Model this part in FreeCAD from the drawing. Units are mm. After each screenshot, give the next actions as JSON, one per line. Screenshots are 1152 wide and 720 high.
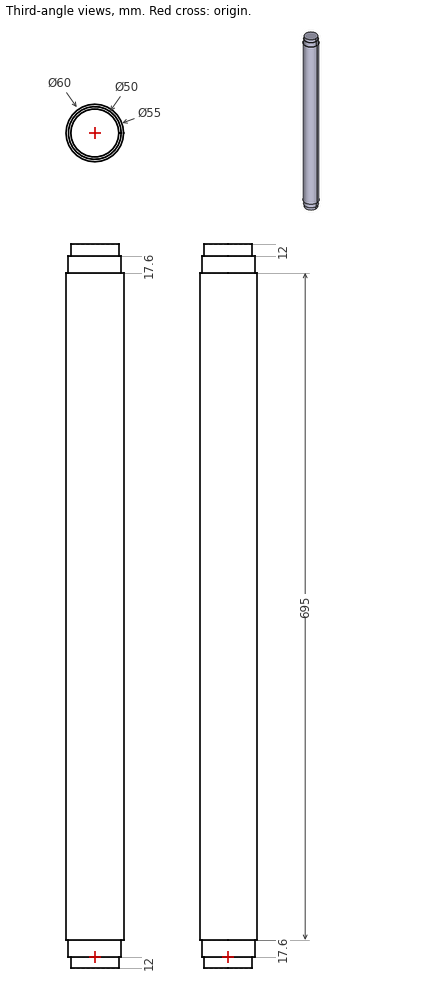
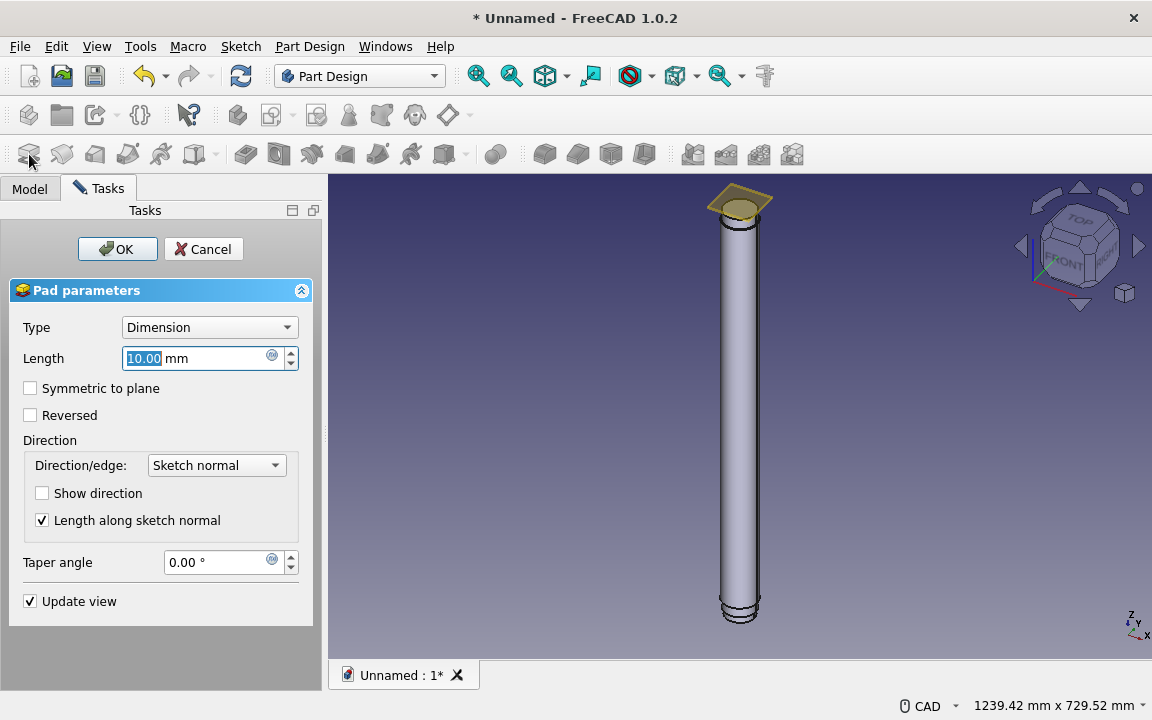
{"action": "type", "text": "12"}
{"action": "key", "text": "Tab"}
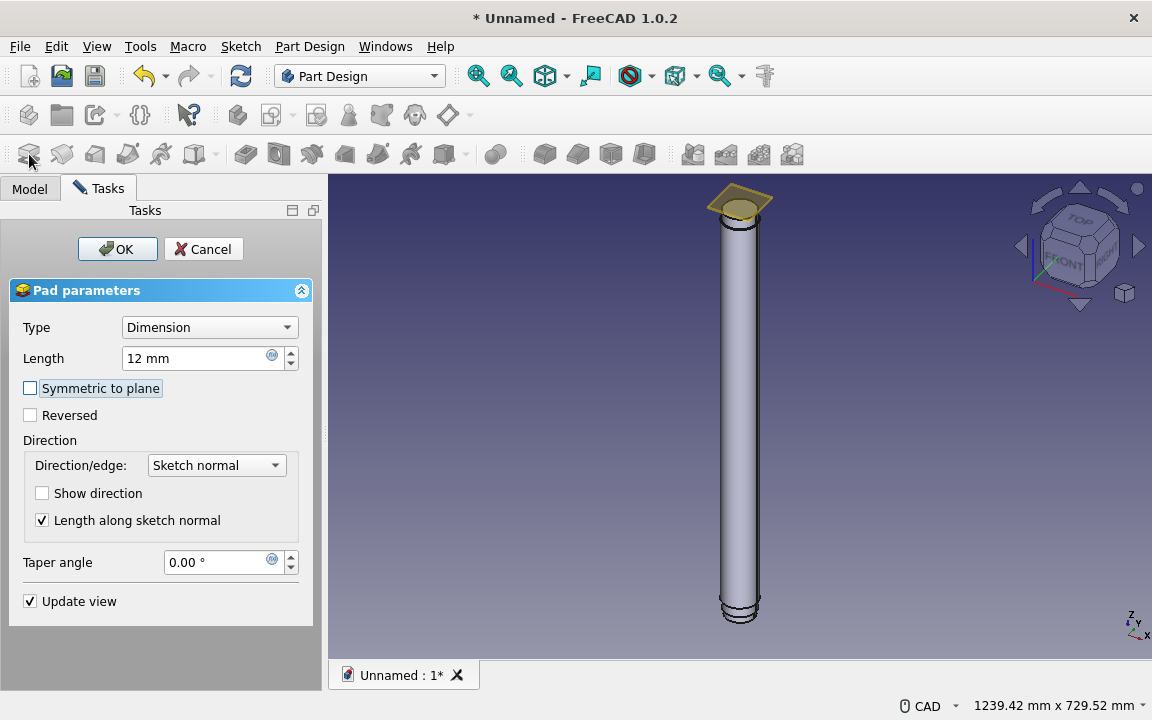
{"action": "left_click", "coordinate": [31, 415]}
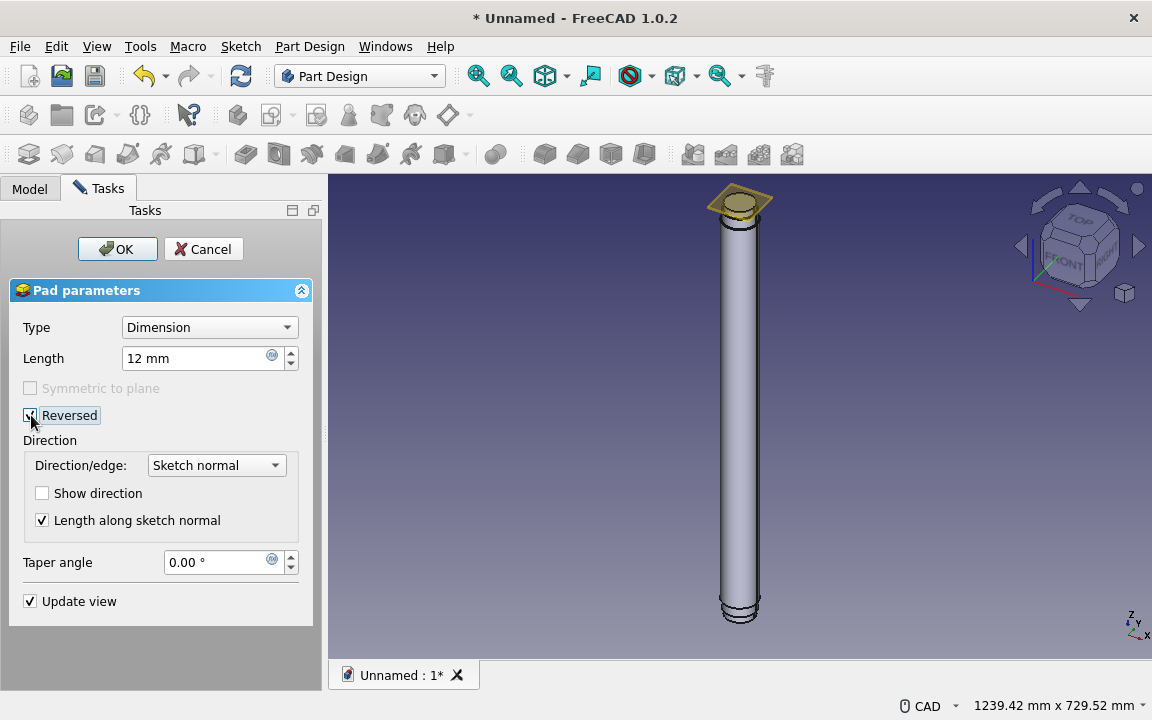
{"action": "left_click", "coordinate": [118, 249]}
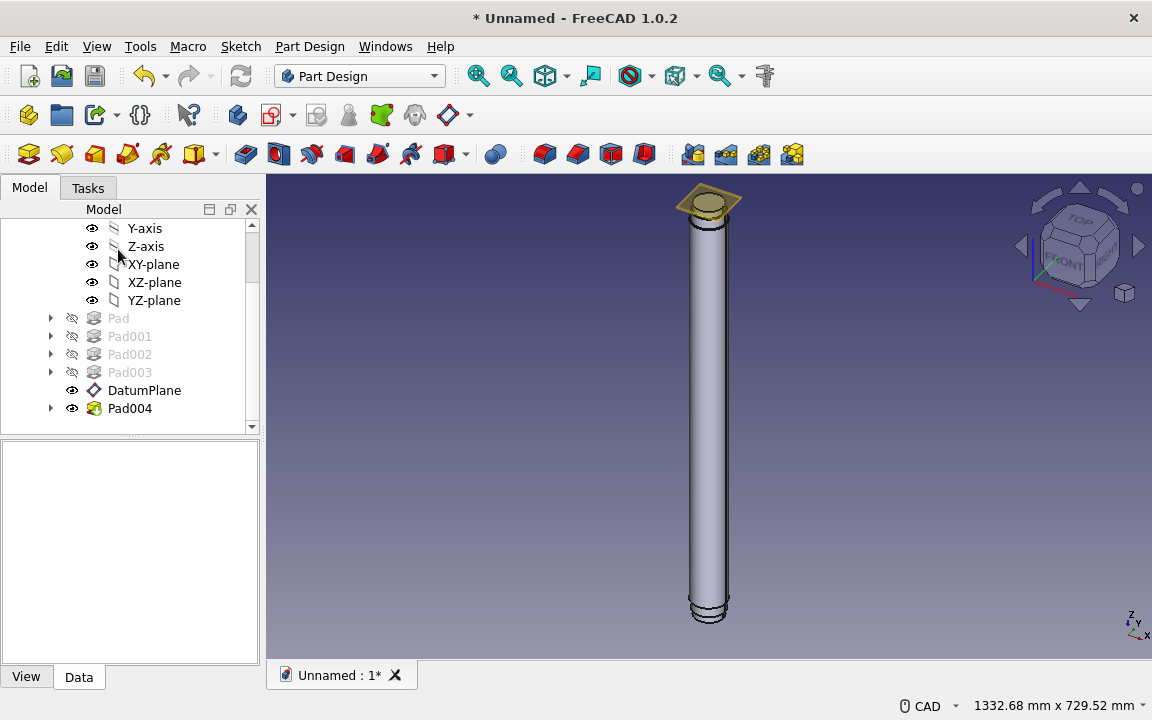
{"action": "left_click", "coordinate": [117, 390]}
{"action": "key", "text": "space"}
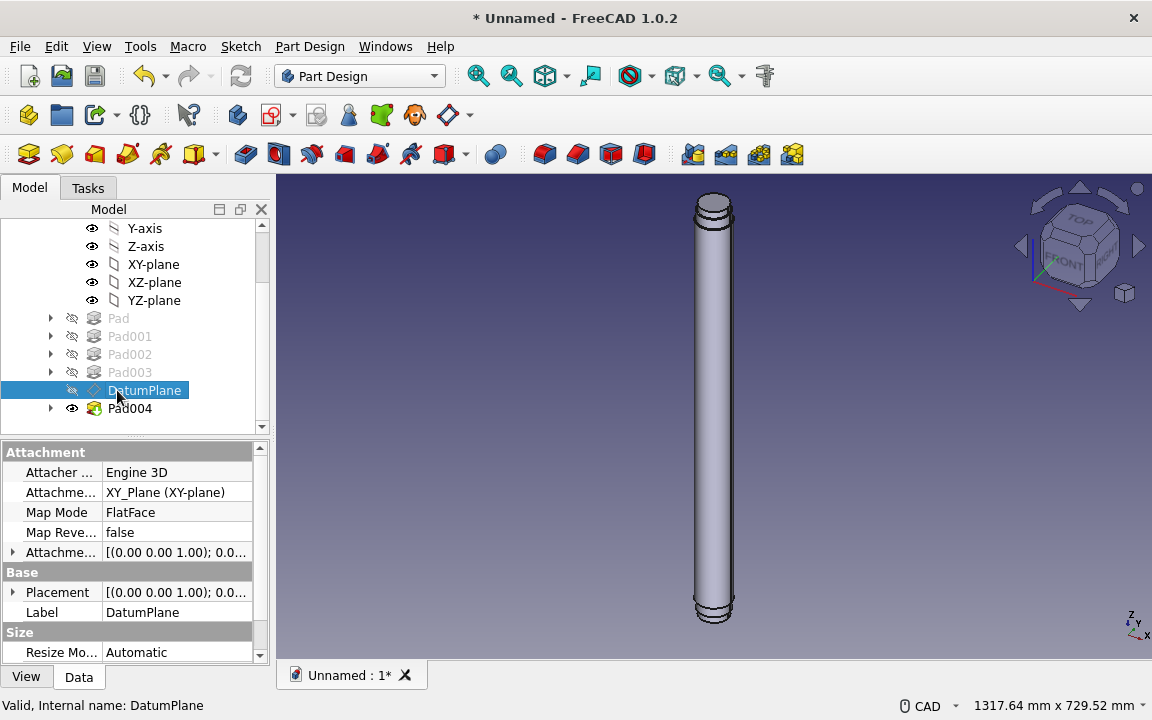
{"action": "key", "text": "0"}